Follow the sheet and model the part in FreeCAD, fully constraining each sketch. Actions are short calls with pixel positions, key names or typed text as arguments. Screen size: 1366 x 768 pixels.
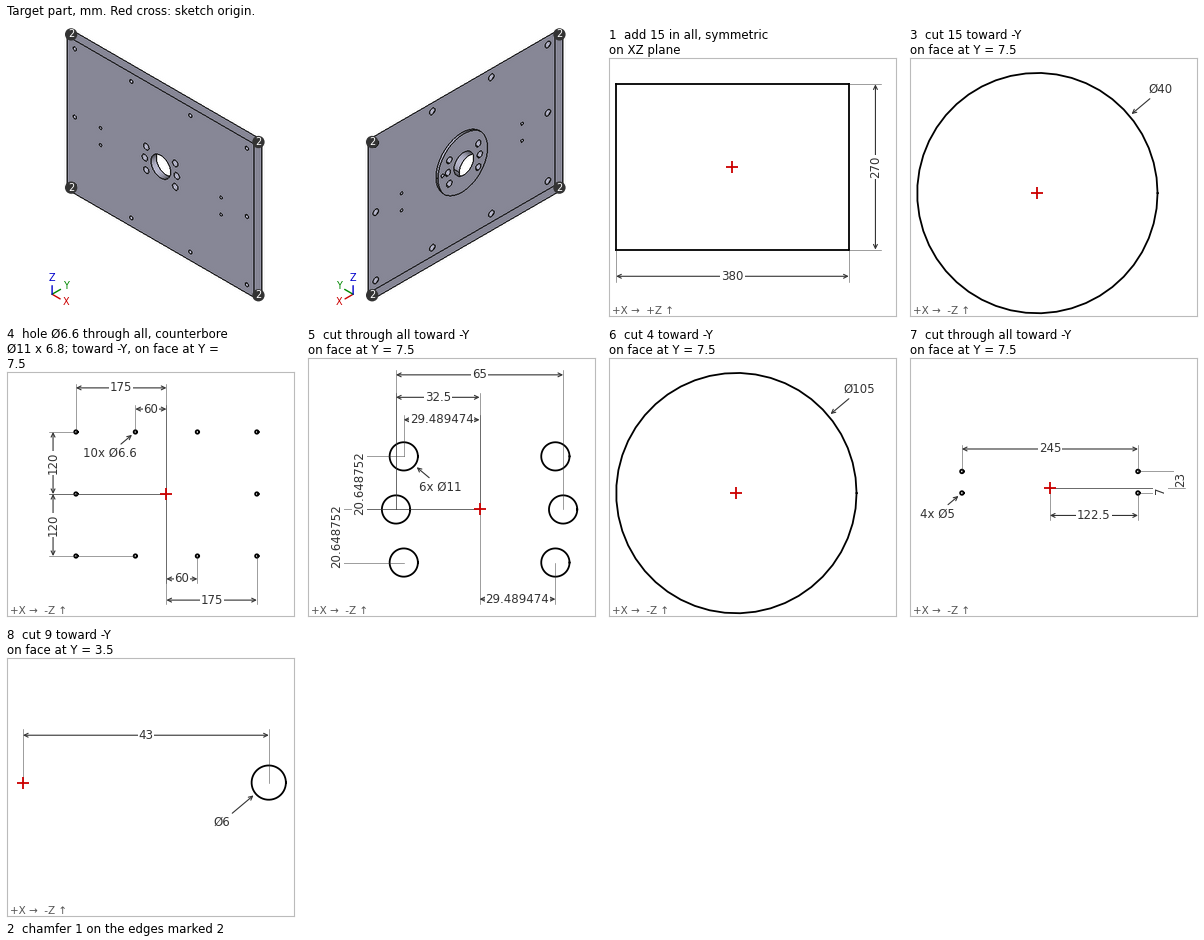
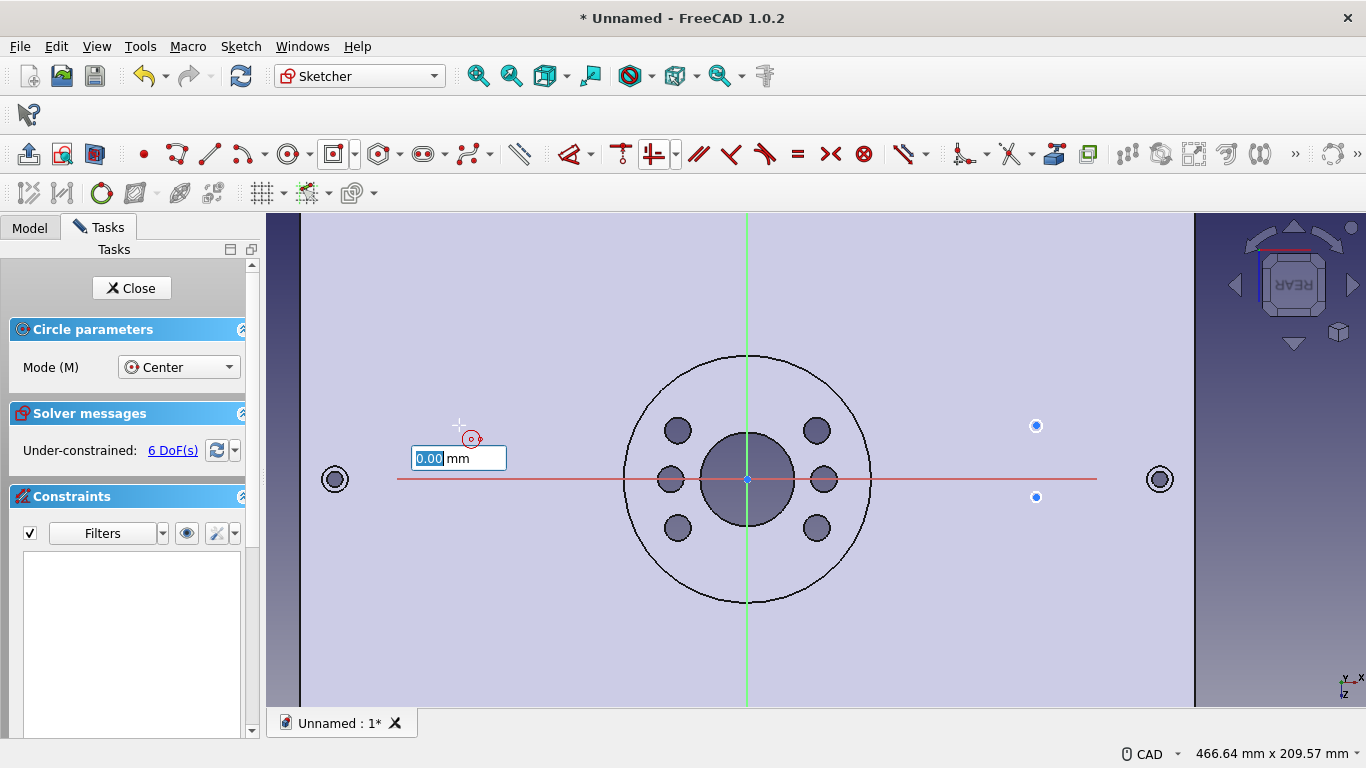
scroll(463, 421, up, 5)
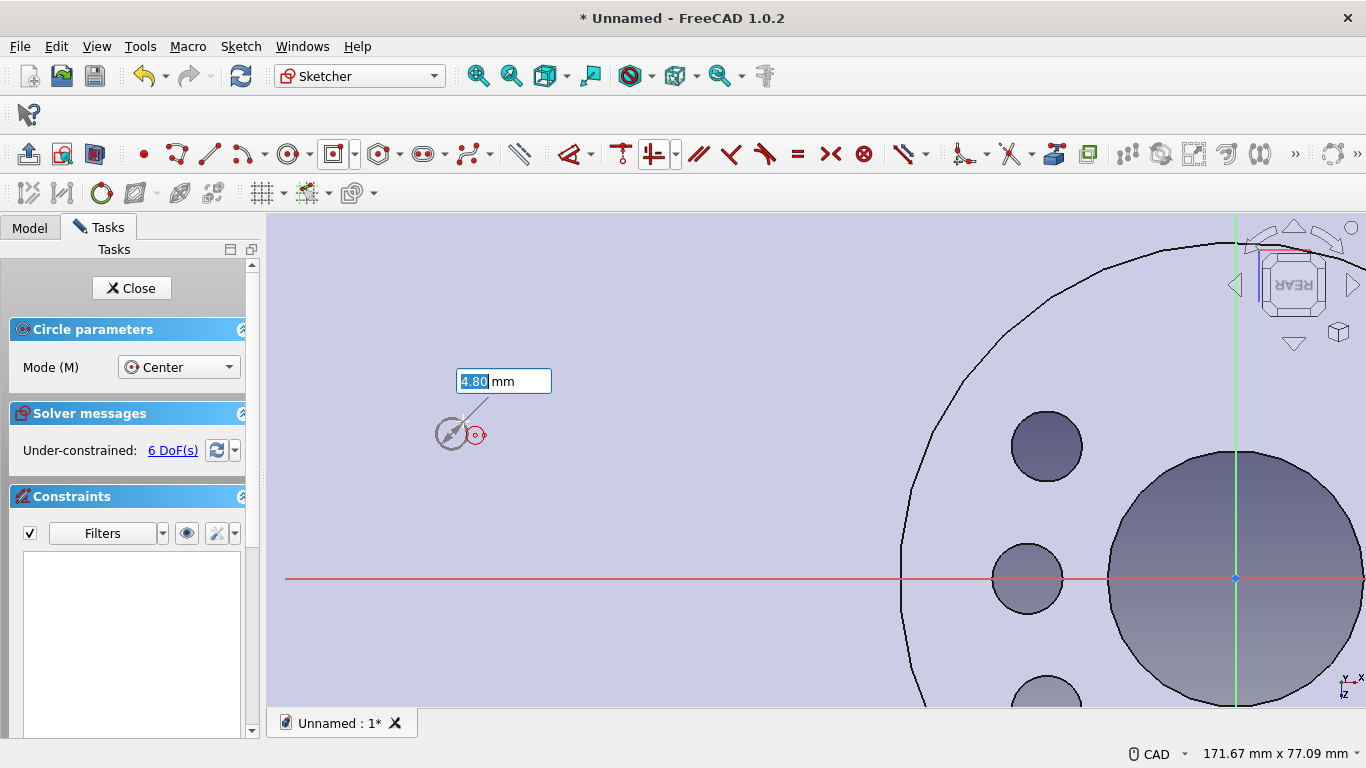
click(462, 420)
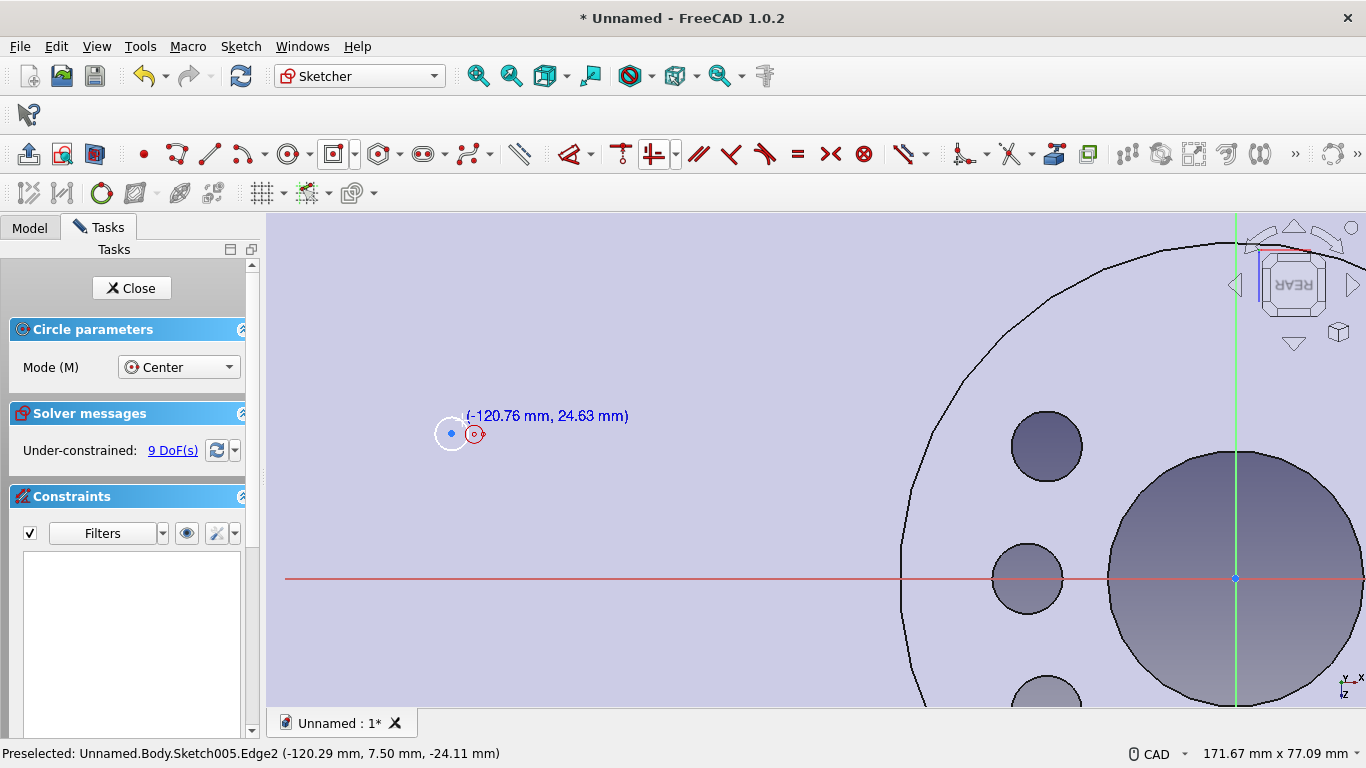
scroll(451, 624, up, 2)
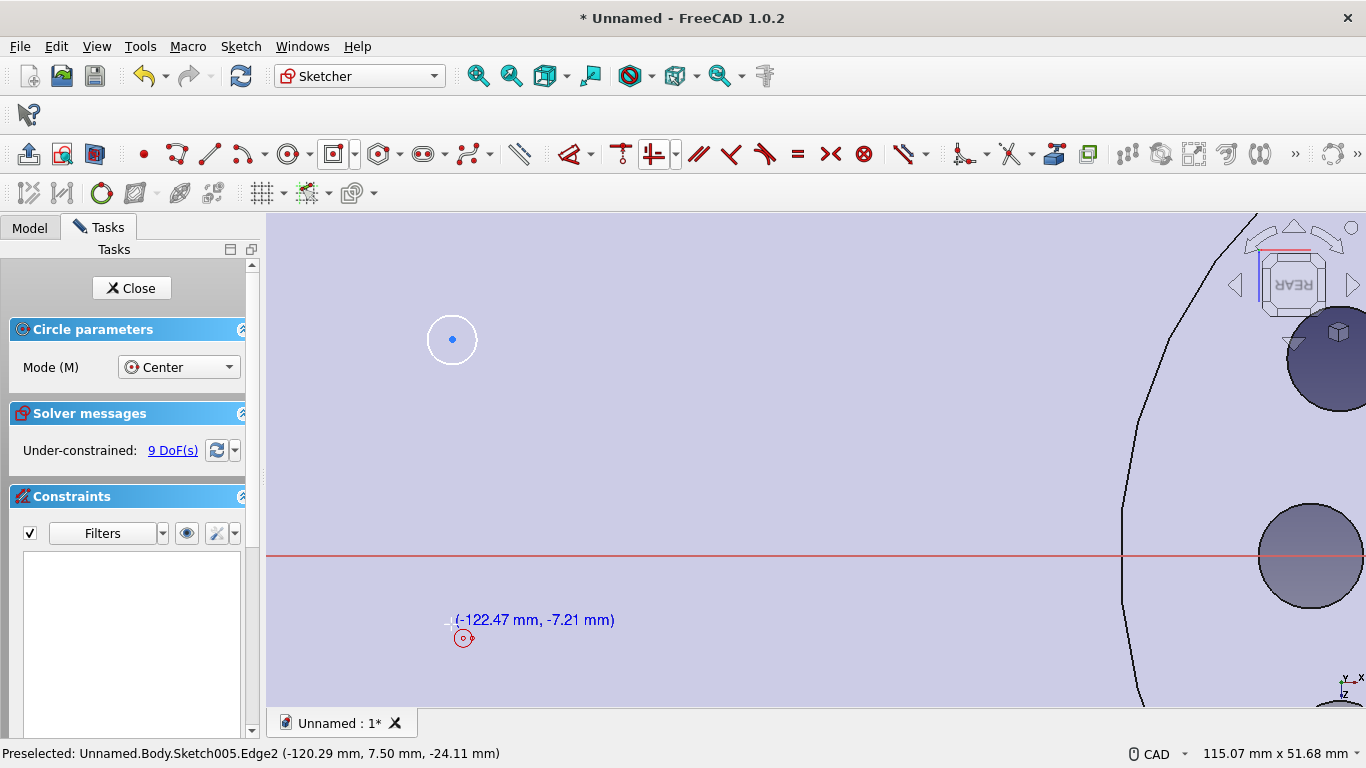
scroll(461, 454, down, 7)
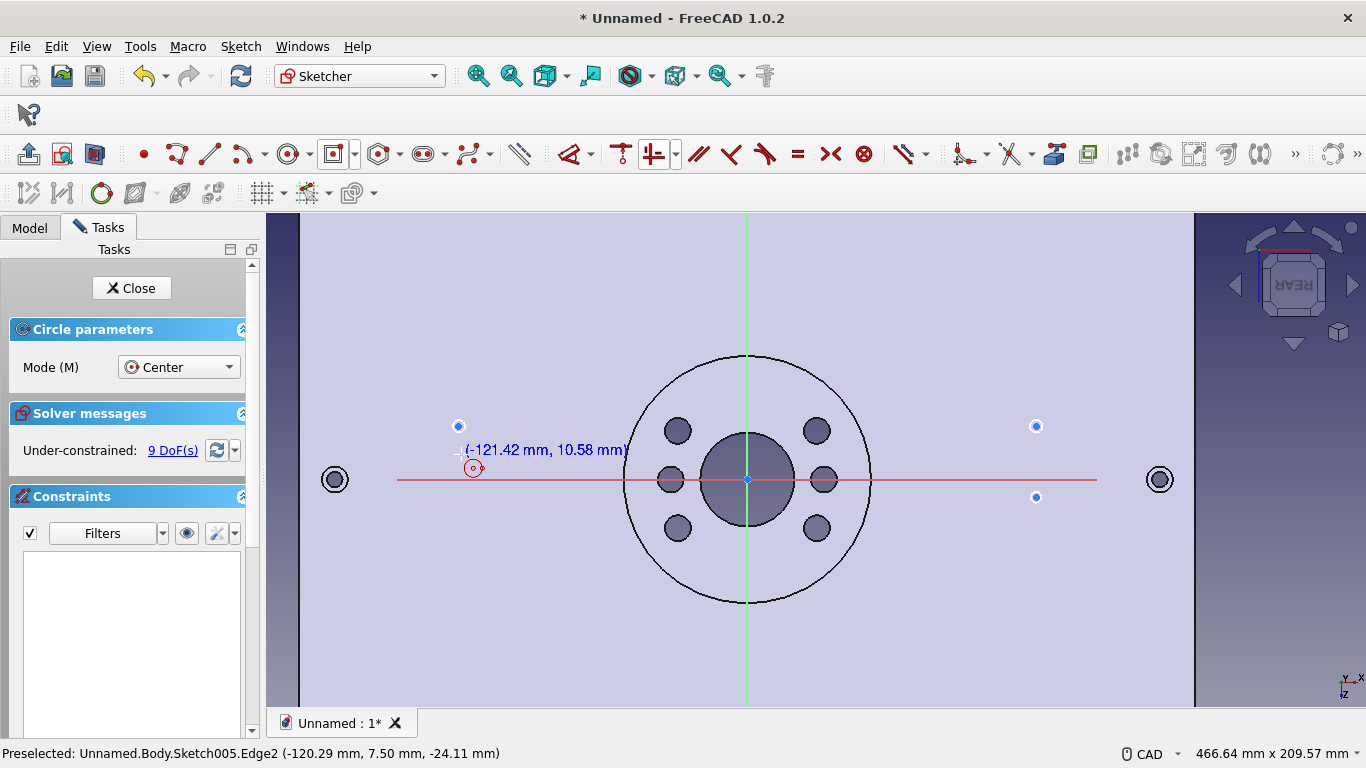
click(459, 496)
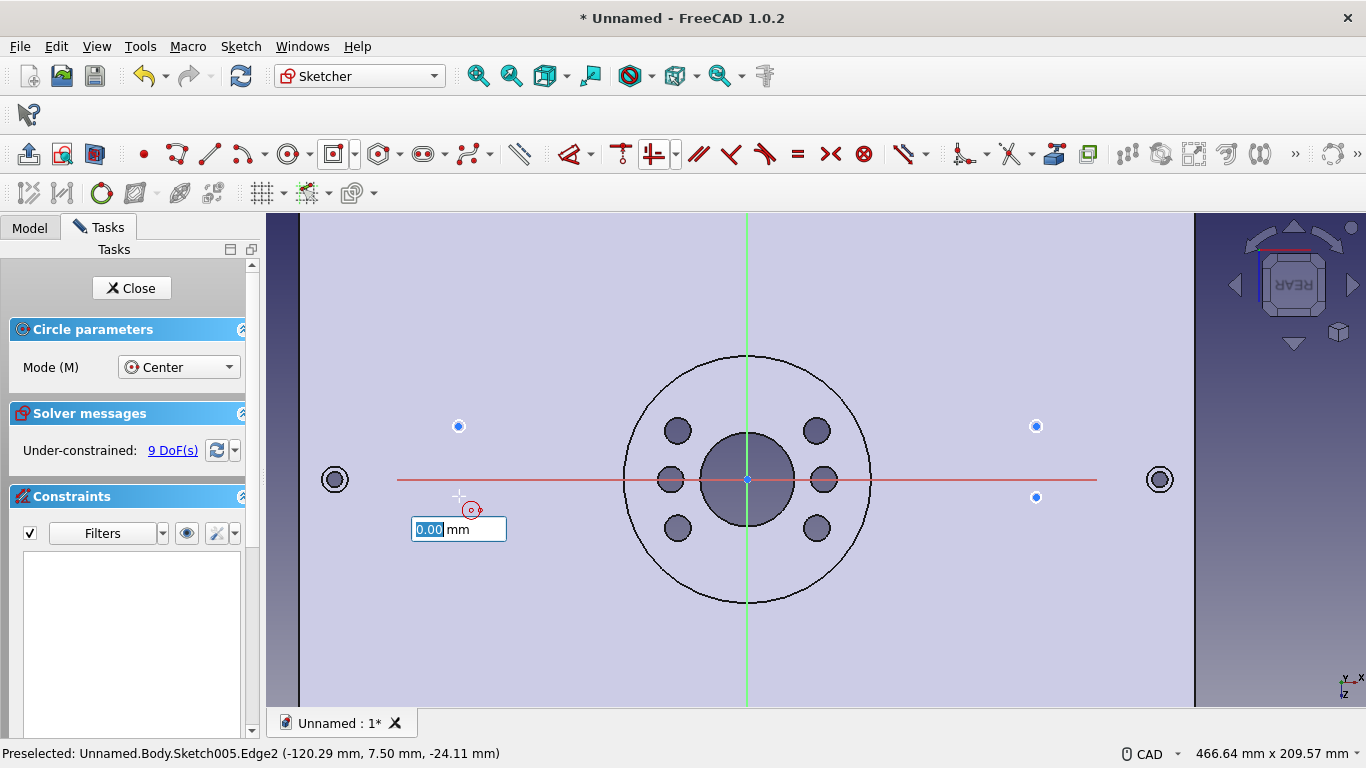
scroll(463, 500, up, 5)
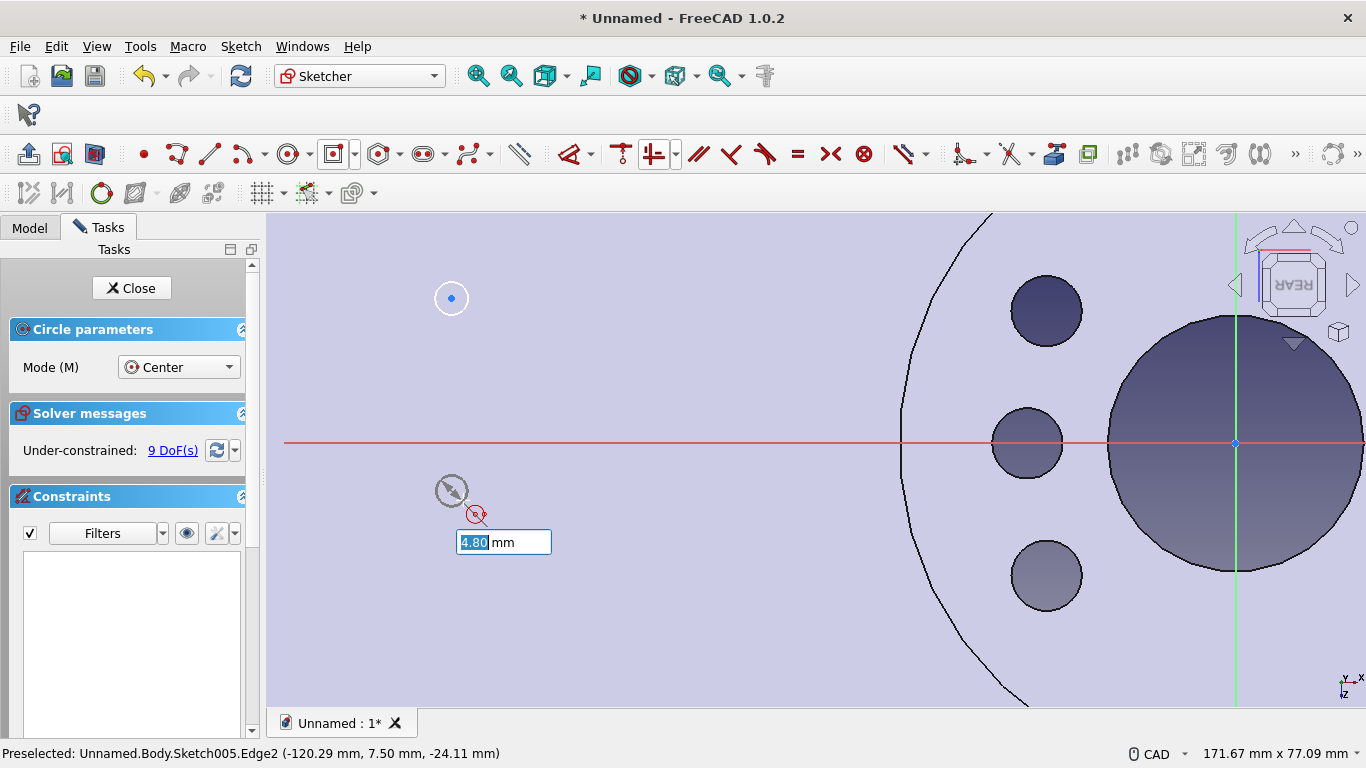
click(462, 500)
key(Escape)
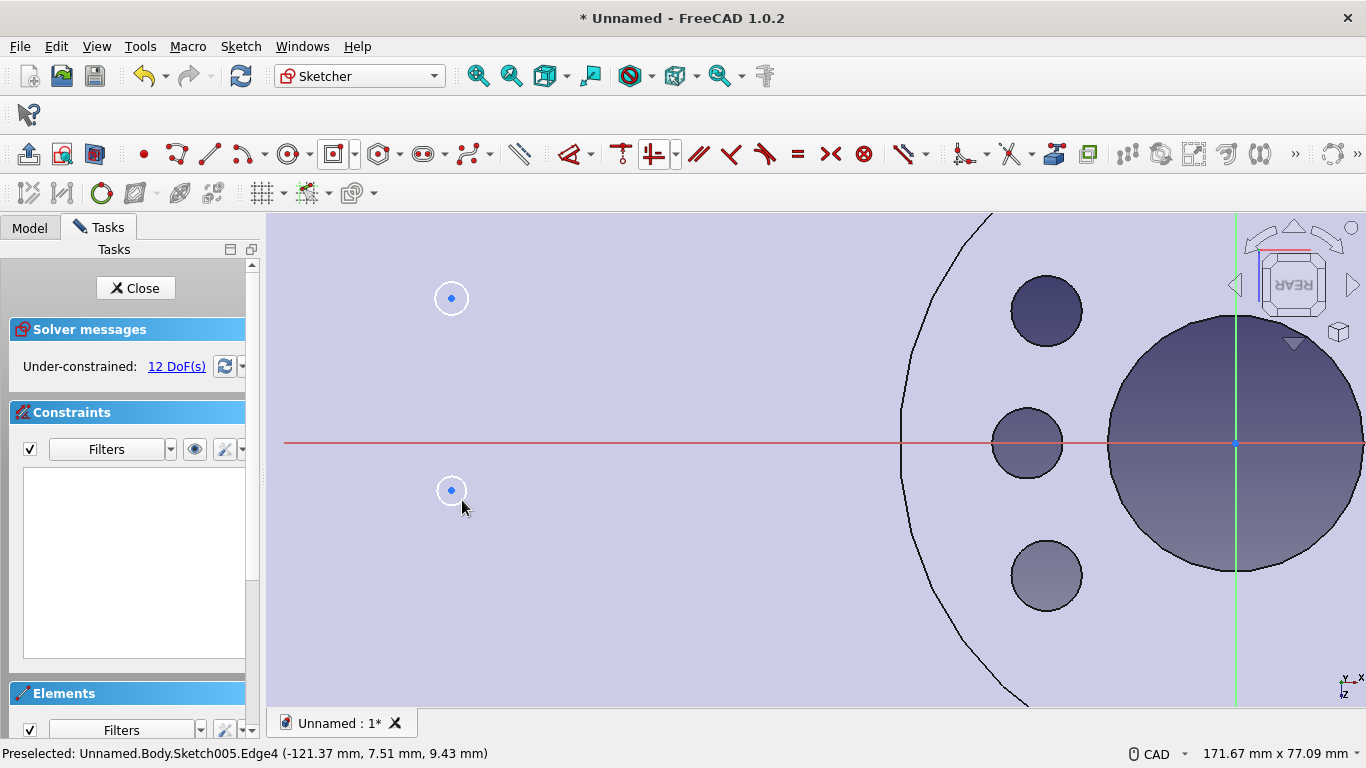
scroll(463, 499, down, 5)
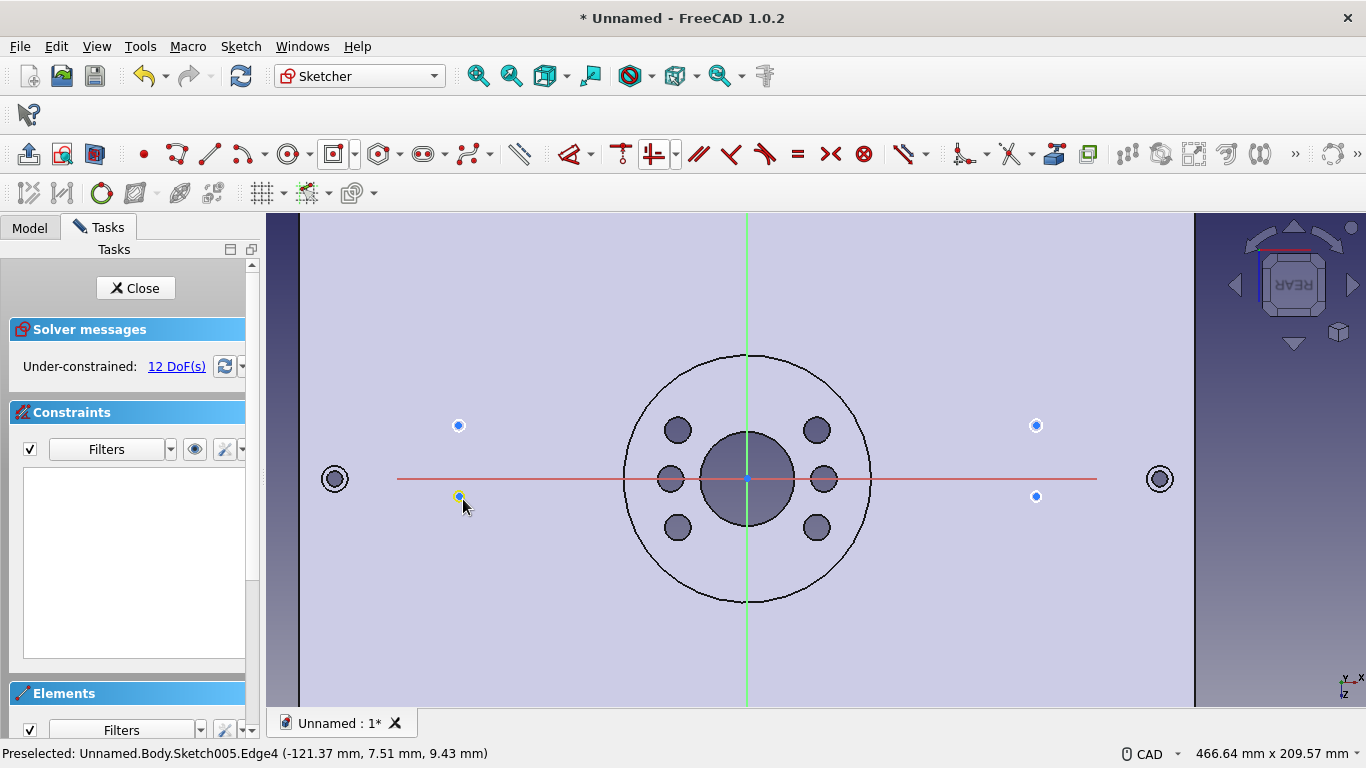
scroll(1040, 493, up, 5)